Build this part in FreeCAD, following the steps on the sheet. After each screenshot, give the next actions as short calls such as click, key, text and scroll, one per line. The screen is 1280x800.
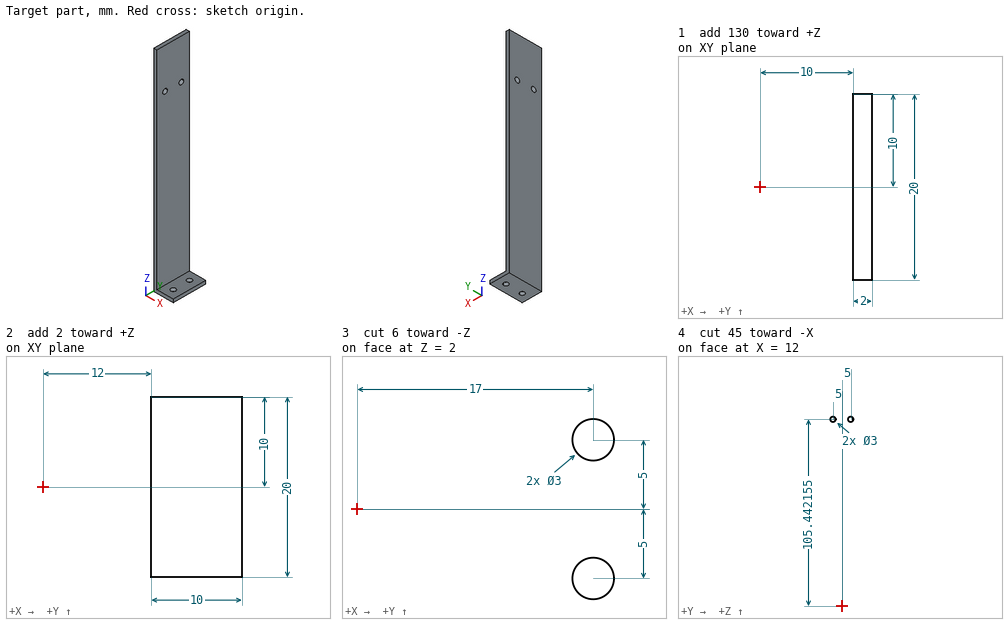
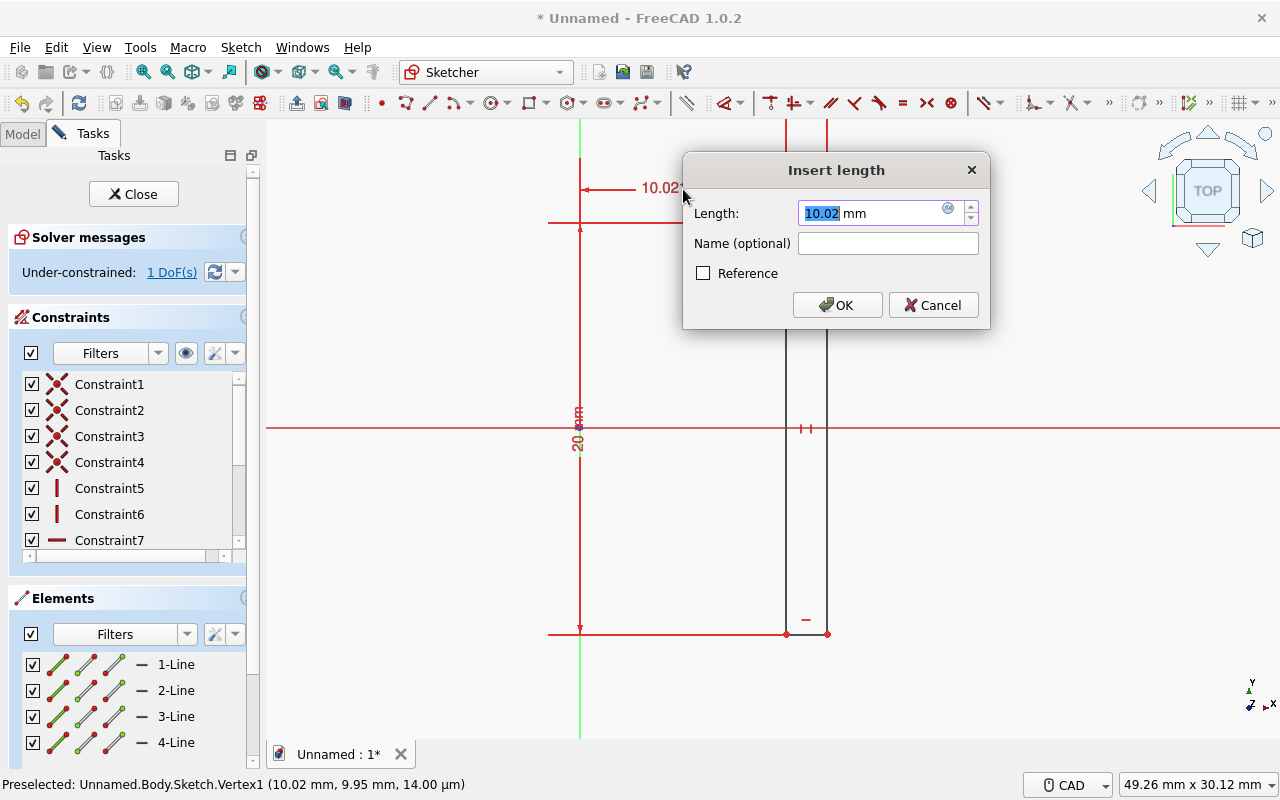
text(10)
key(Return)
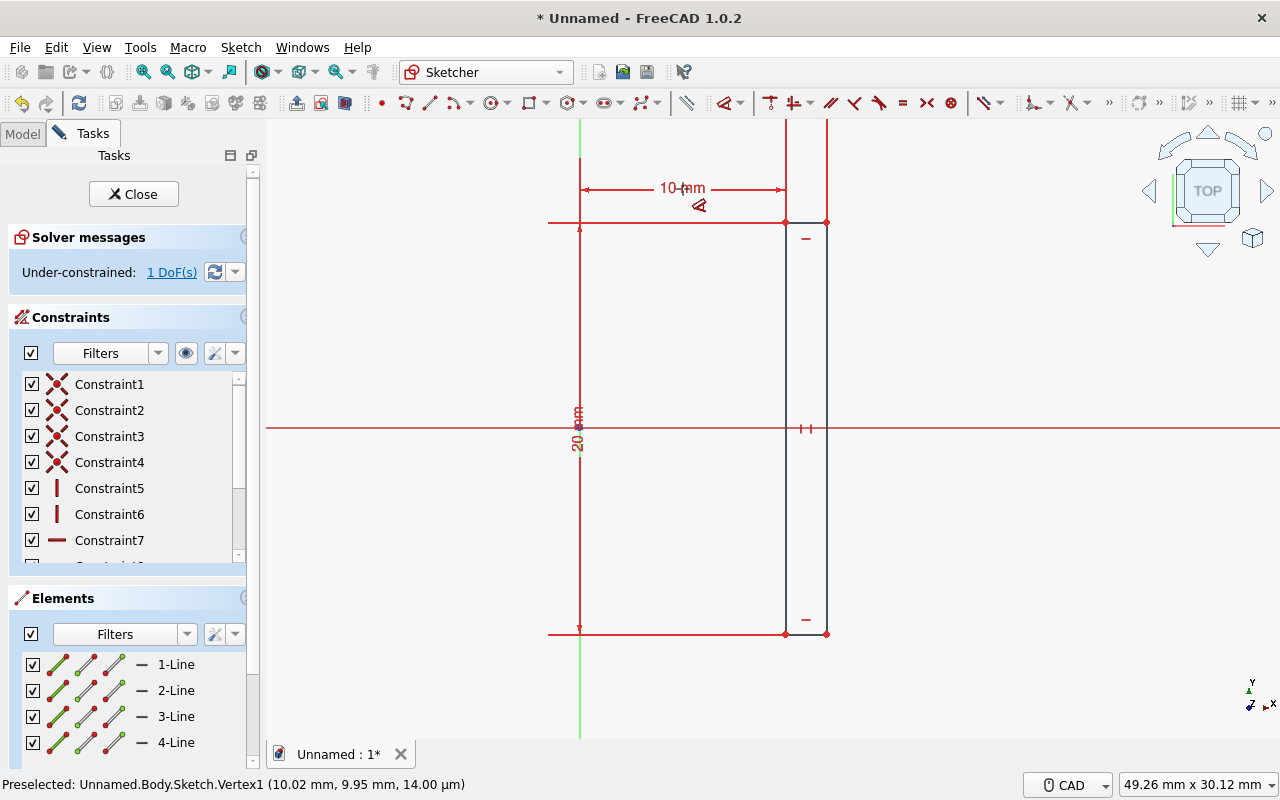
click(786, 223)
click(546, 325)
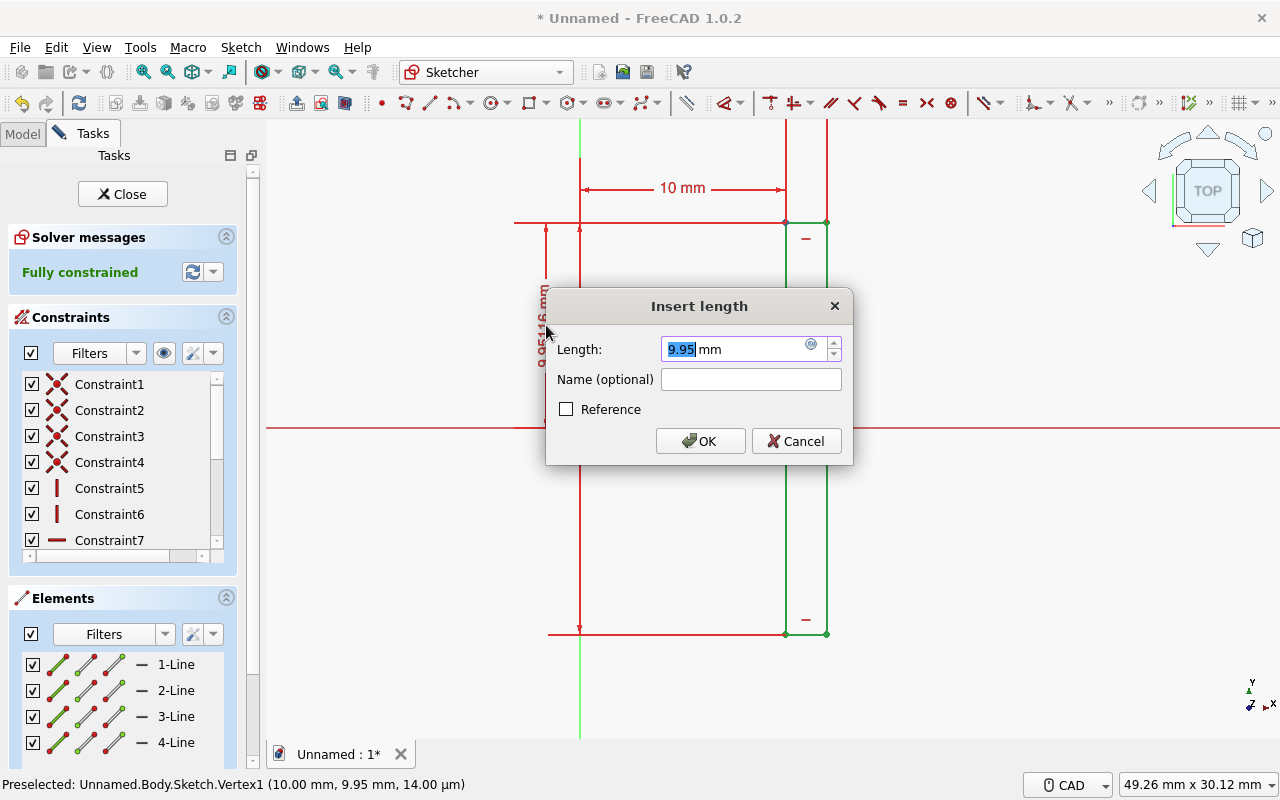
text(10)
key(Return)
key(Escape)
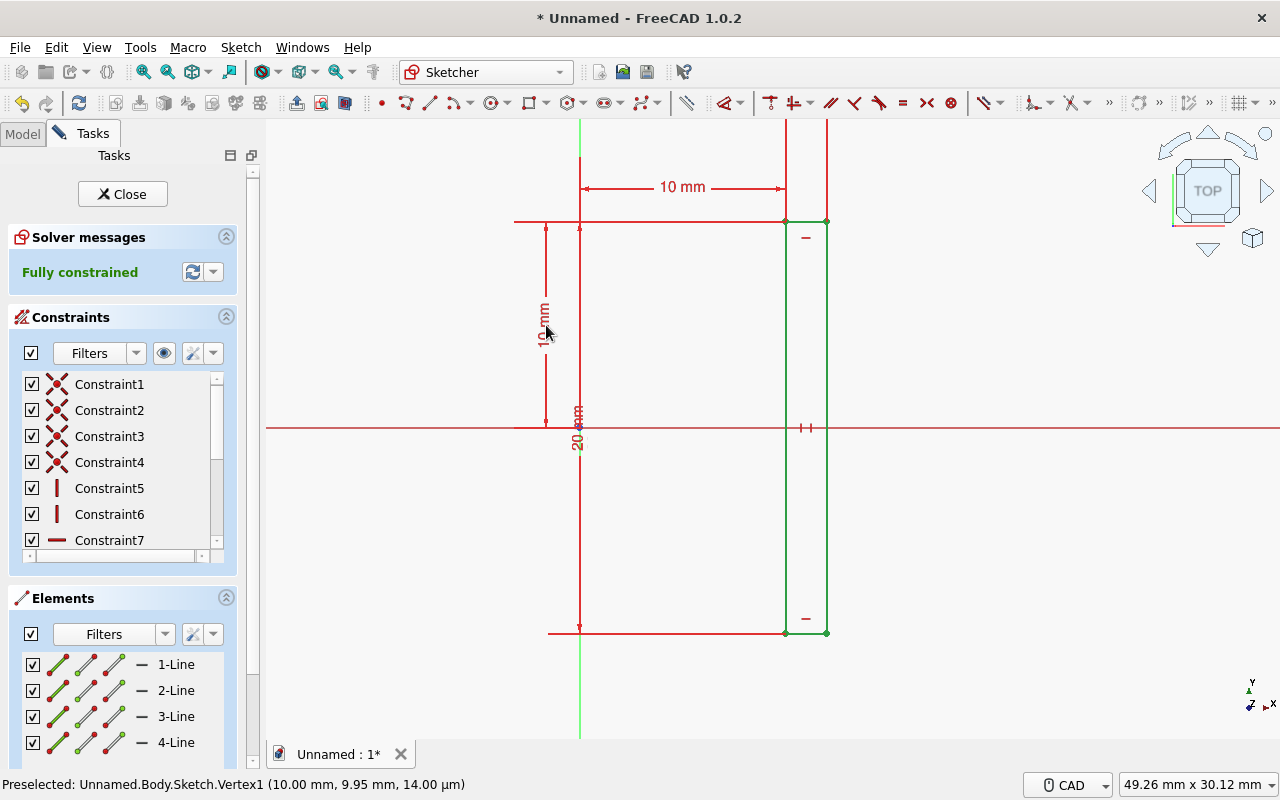
click(123, 194)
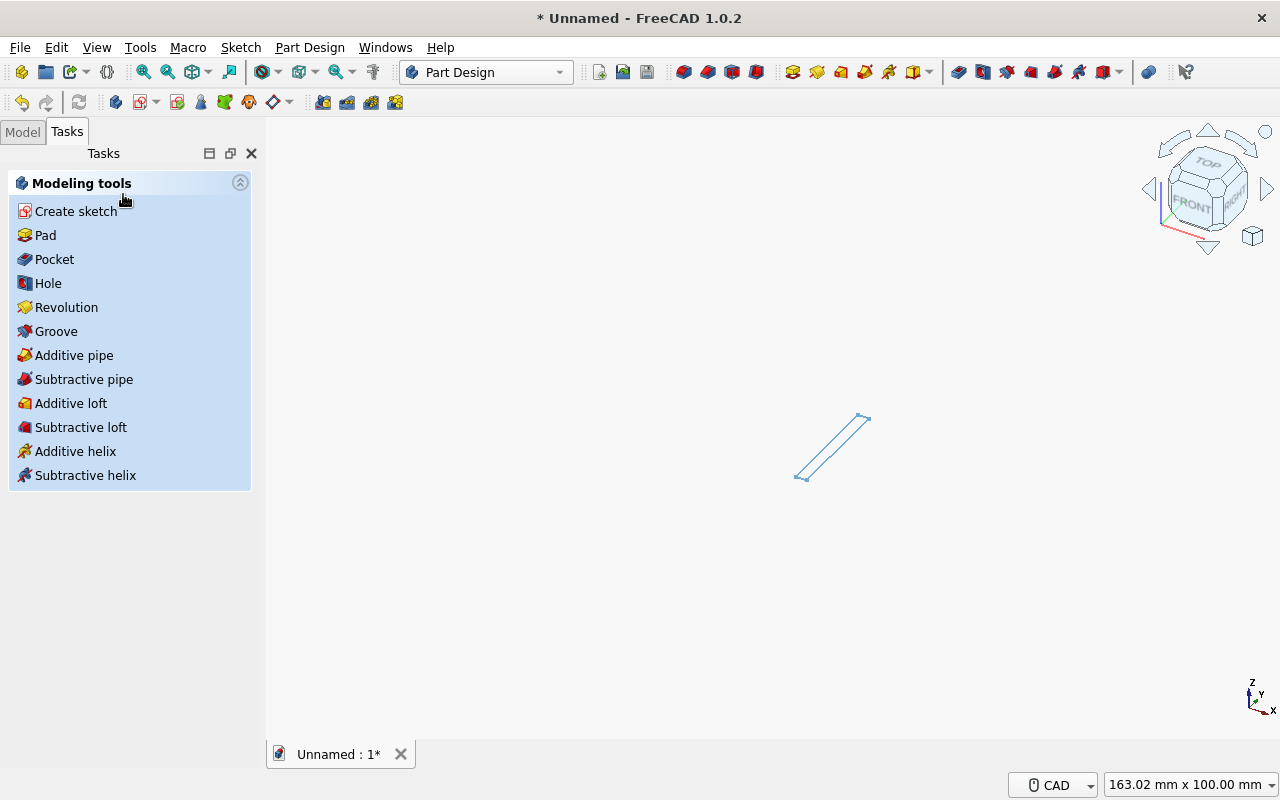
click(794, 72)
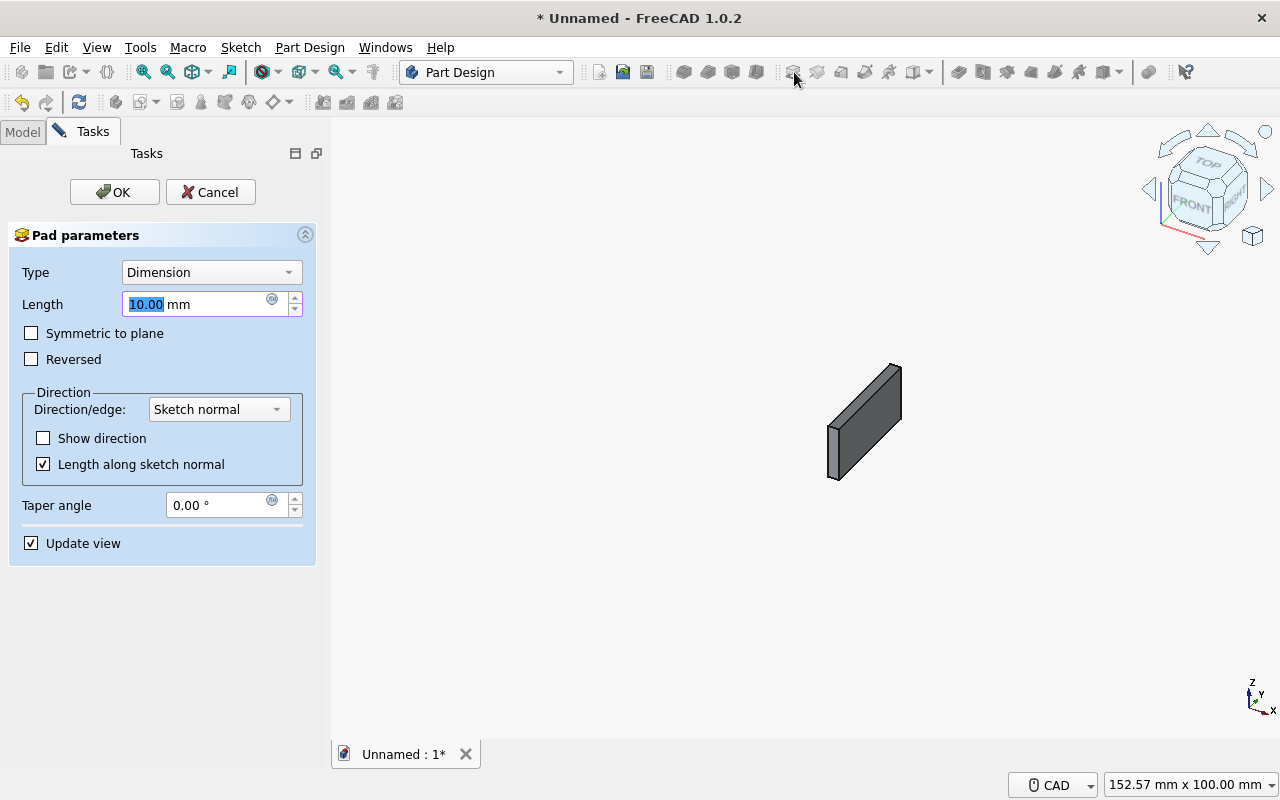
text(130)
key(Tab)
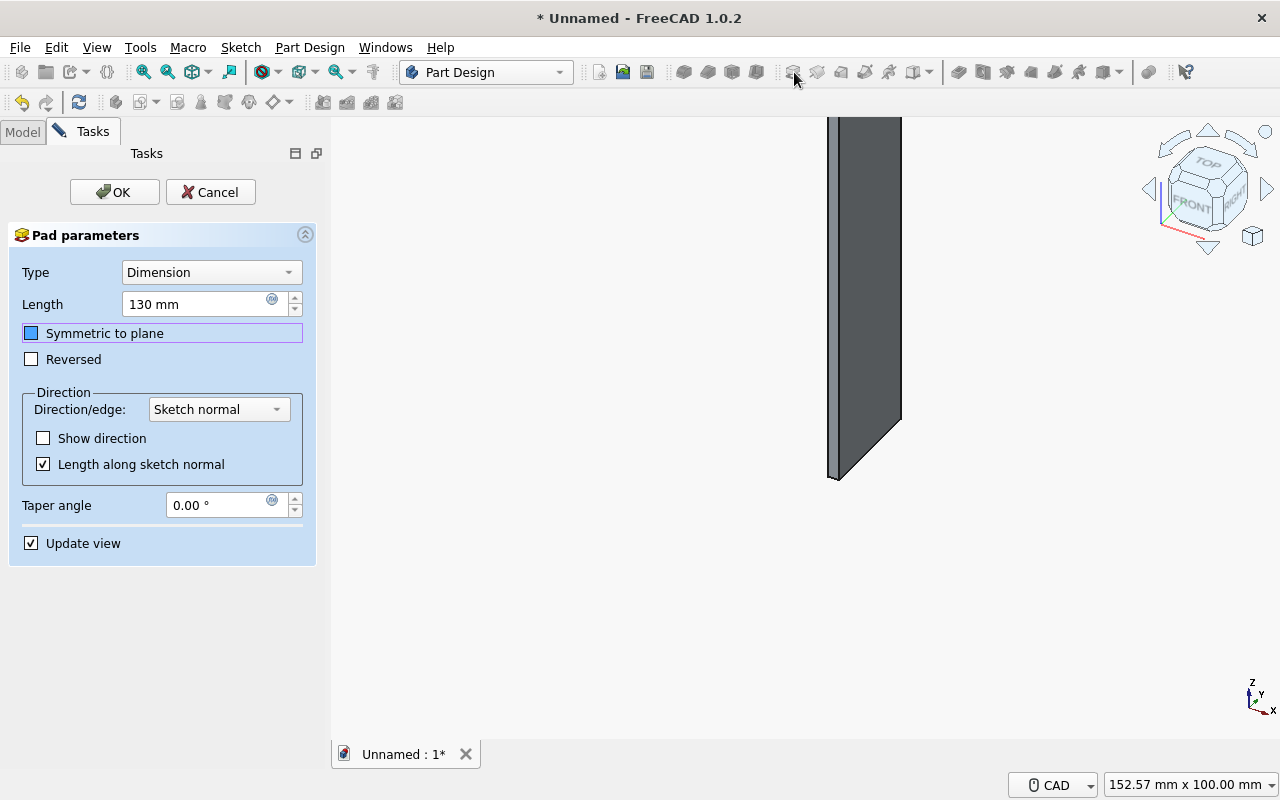
click(115, 192)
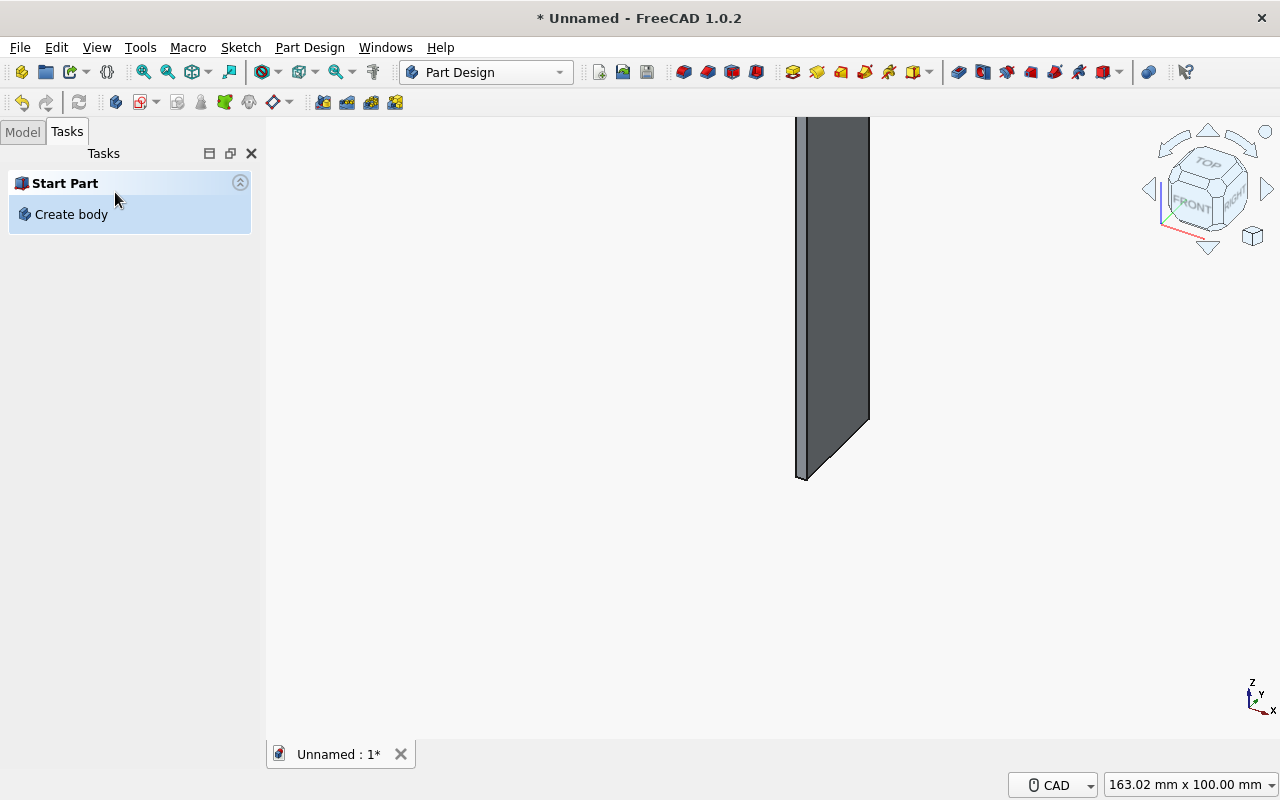
key(v)
key(f)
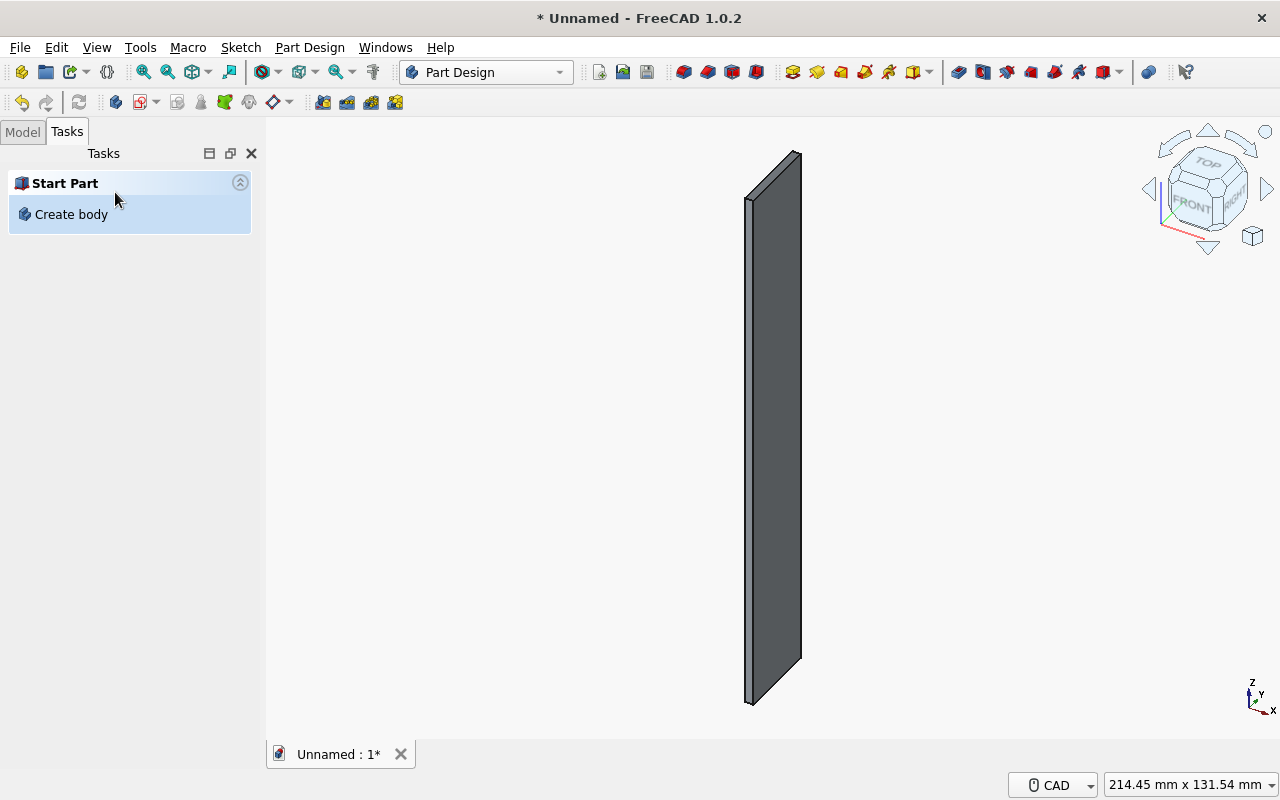
click(140, 102)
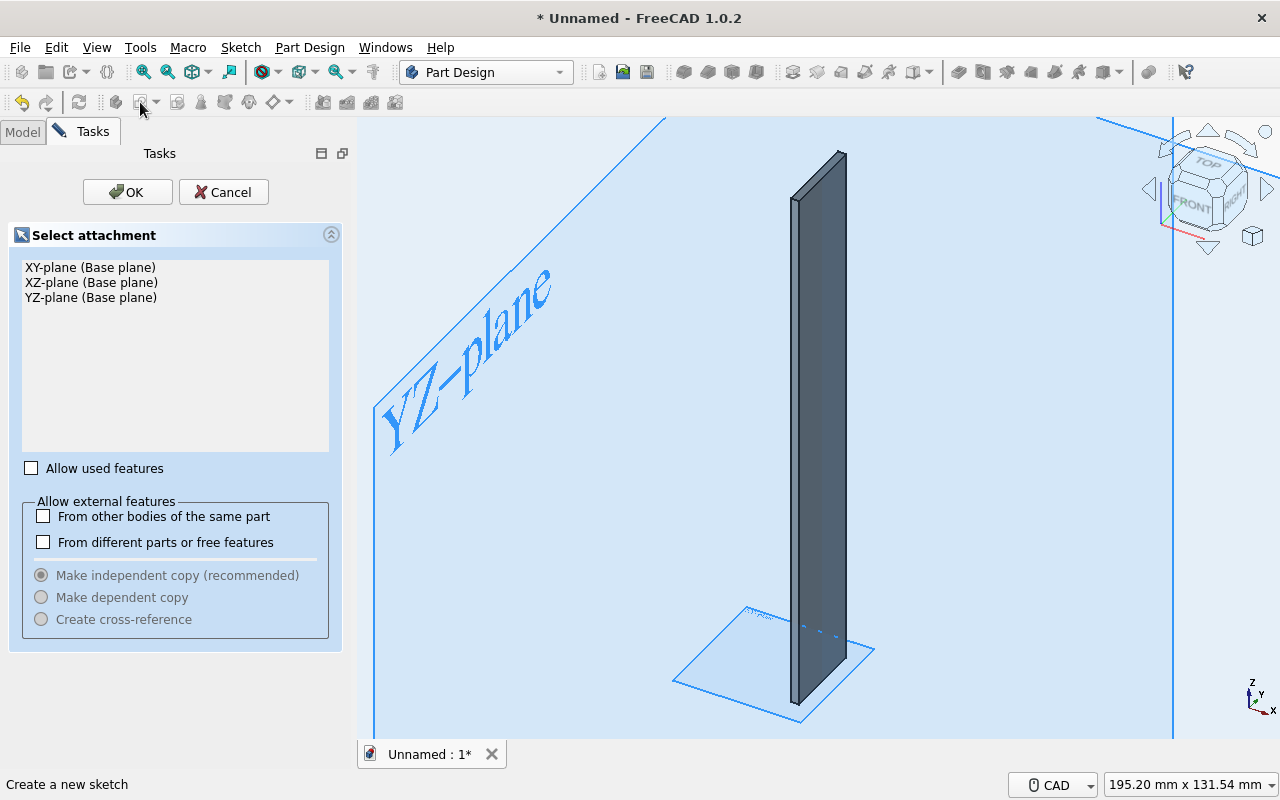
click(82, 268)